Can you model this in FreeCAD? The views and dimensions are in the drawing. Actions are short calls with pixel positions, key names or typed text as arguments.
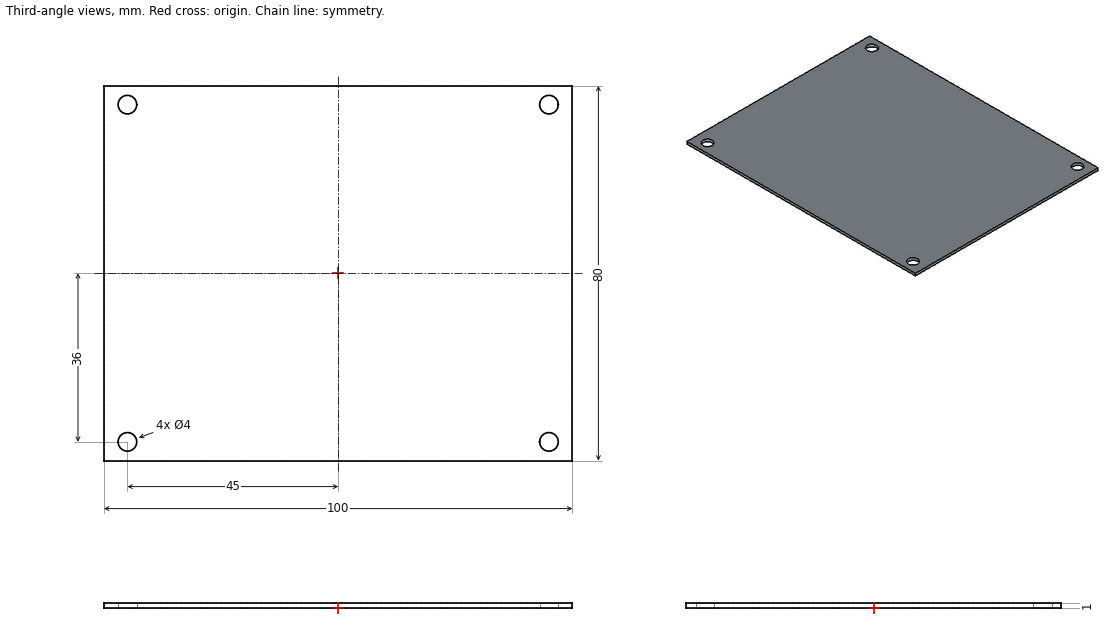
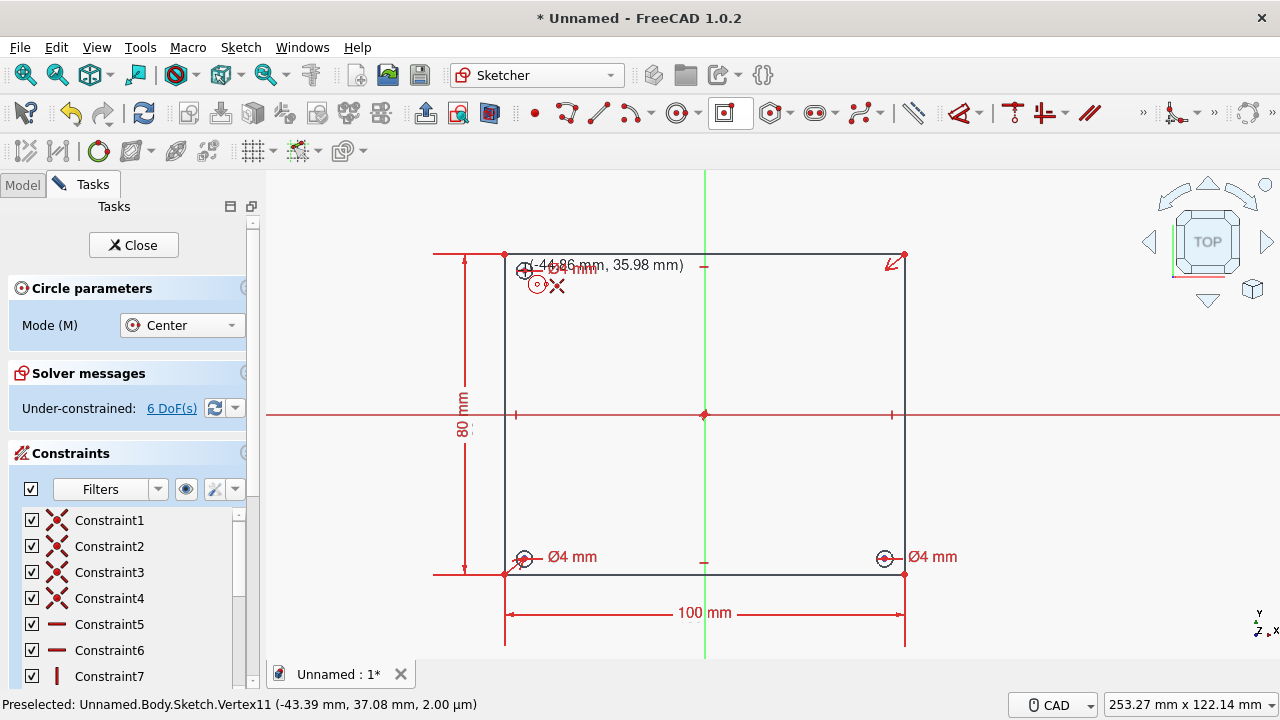
scroll(885, 270, up, 6)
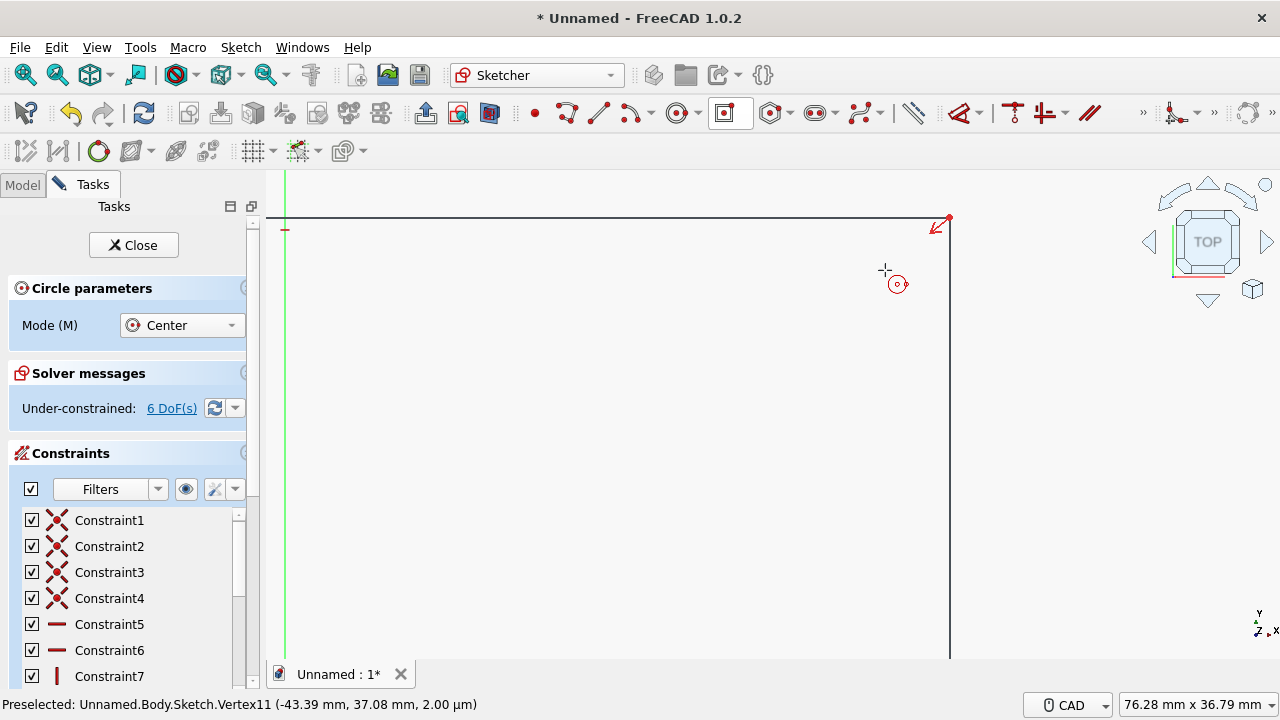
click(883, 271)
move(902, 252)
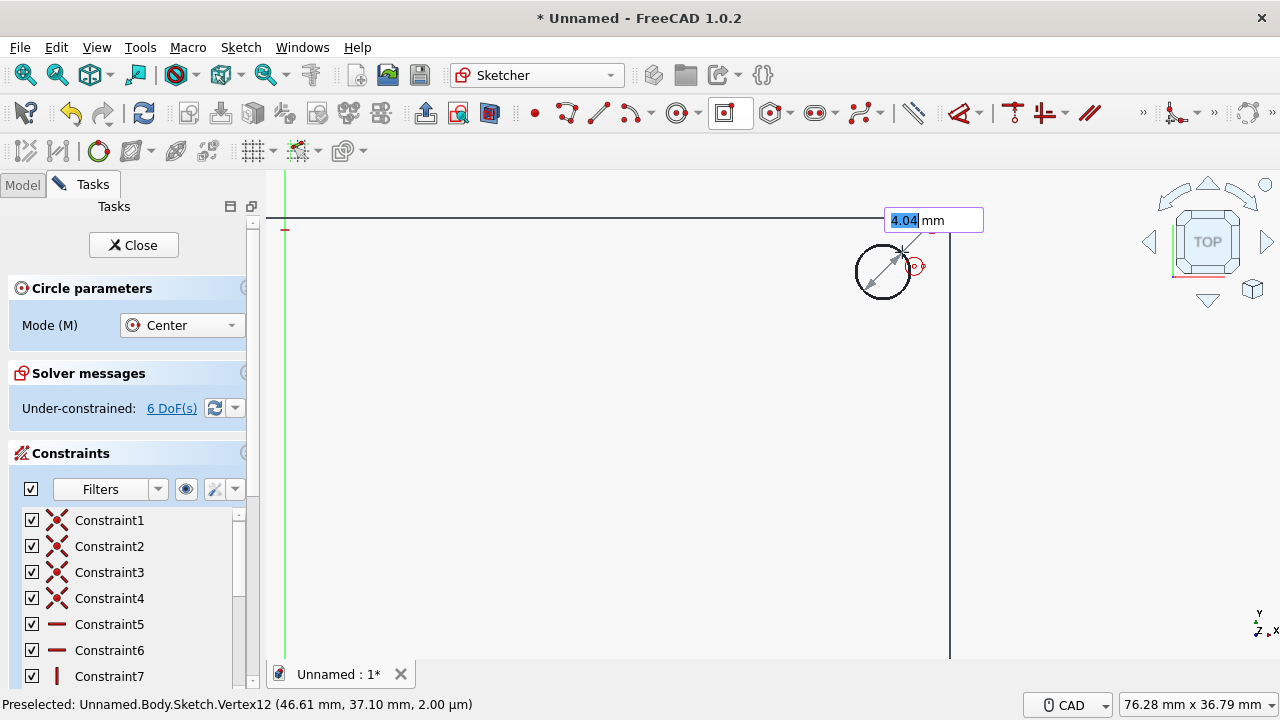
text(4)
key(Return)
key(Escape)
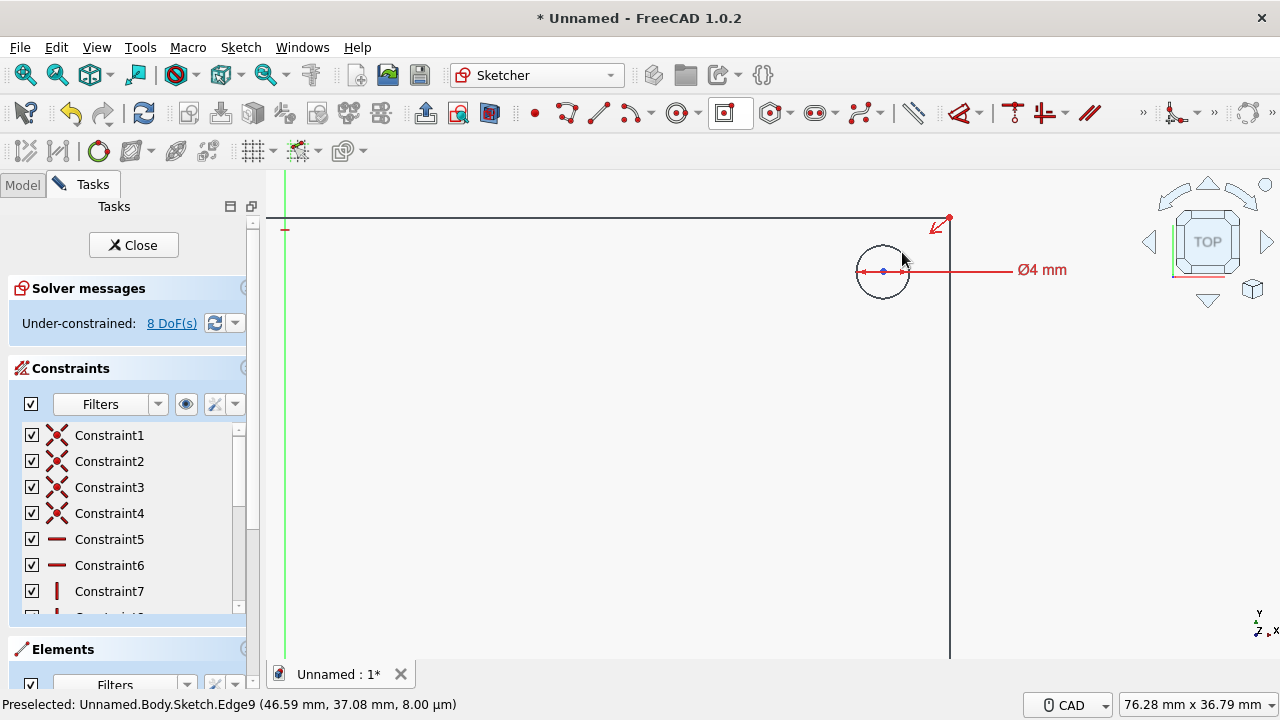
scroll(885, 270, down, 6)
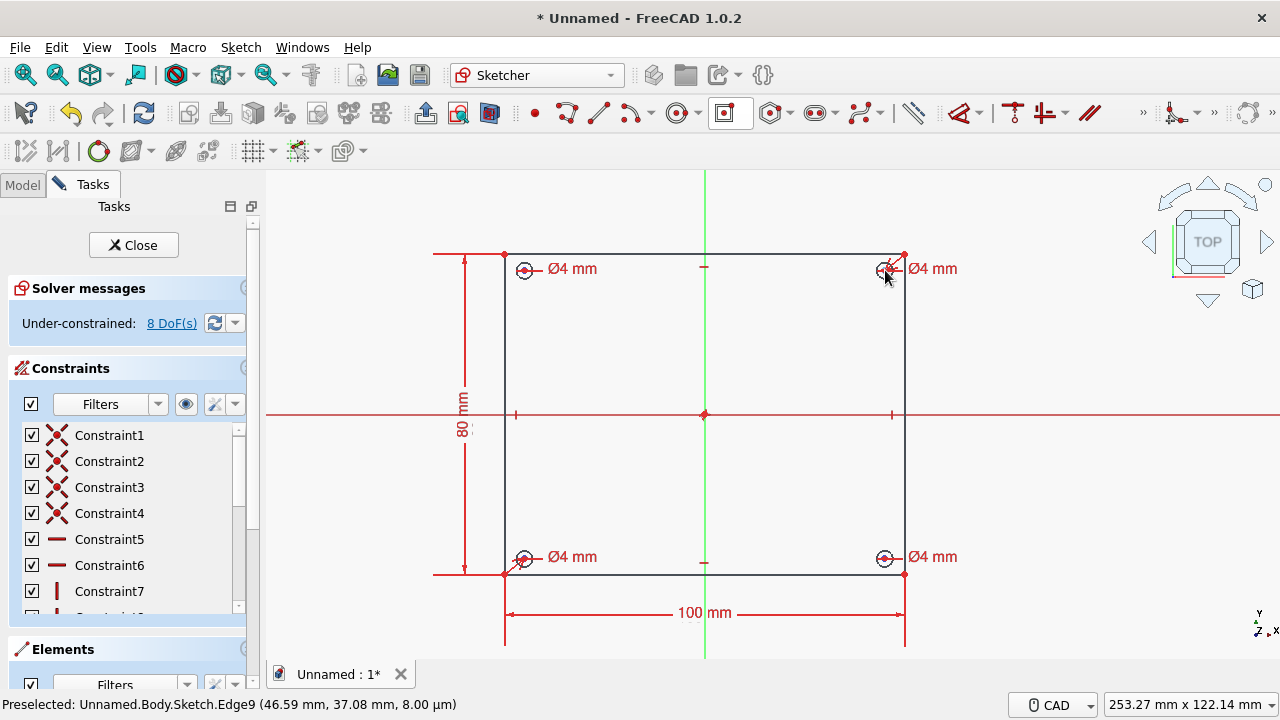
click(525, 559)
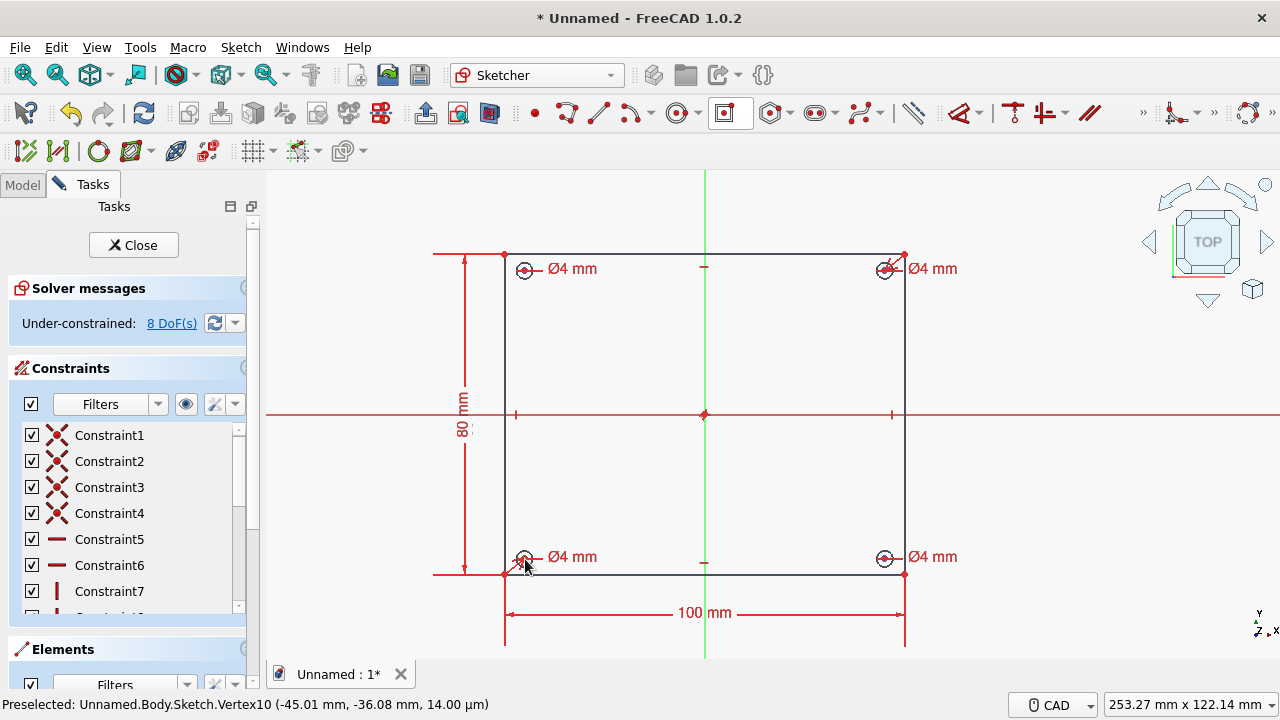
click(885, 559)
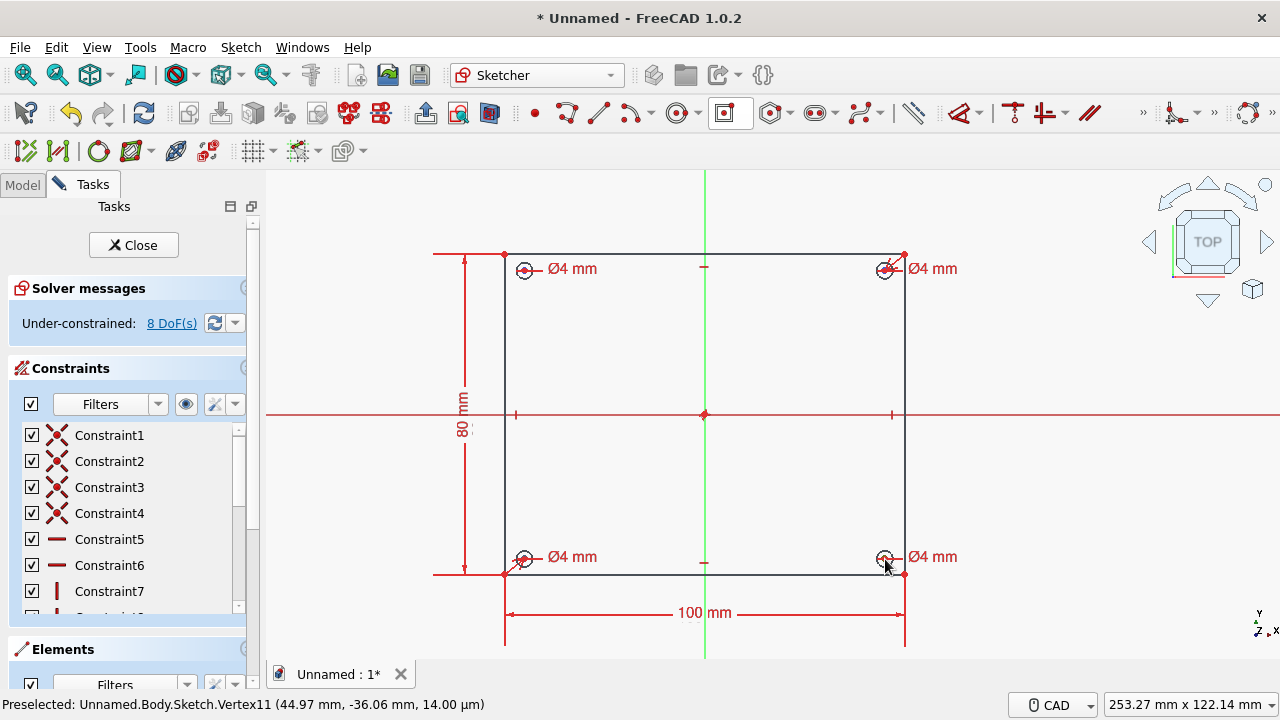
click(705, 538)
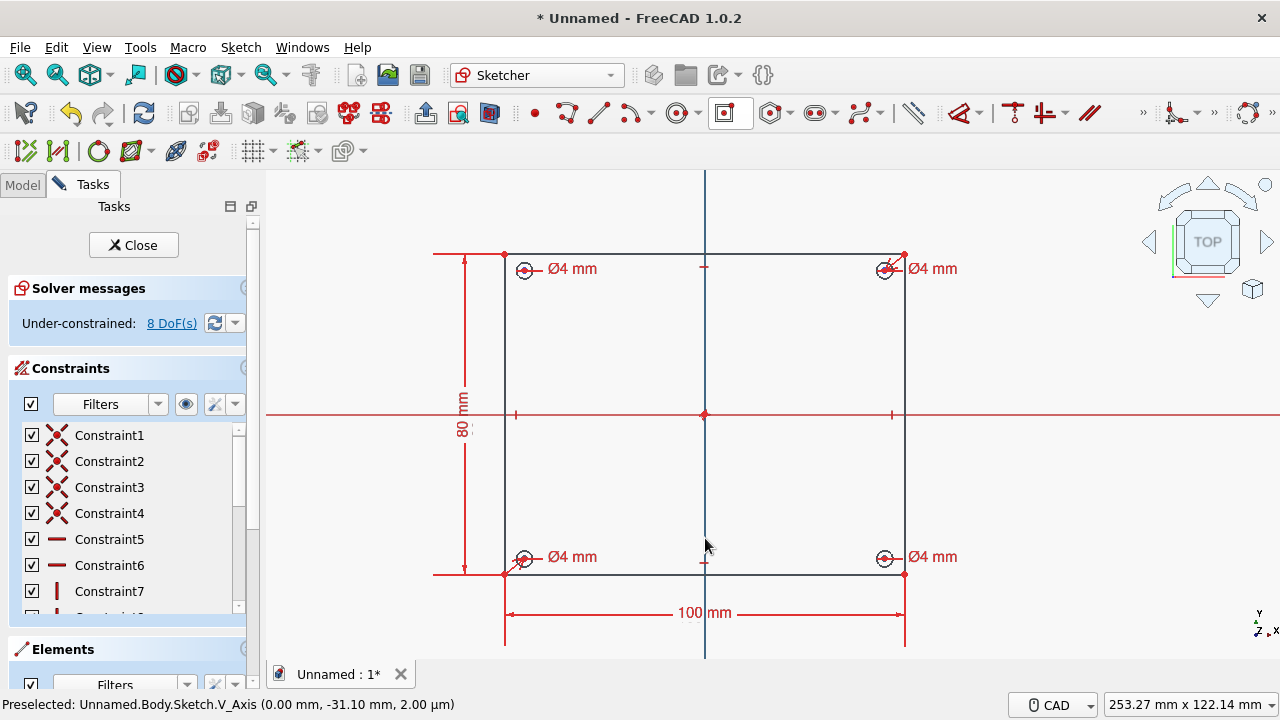
key(s)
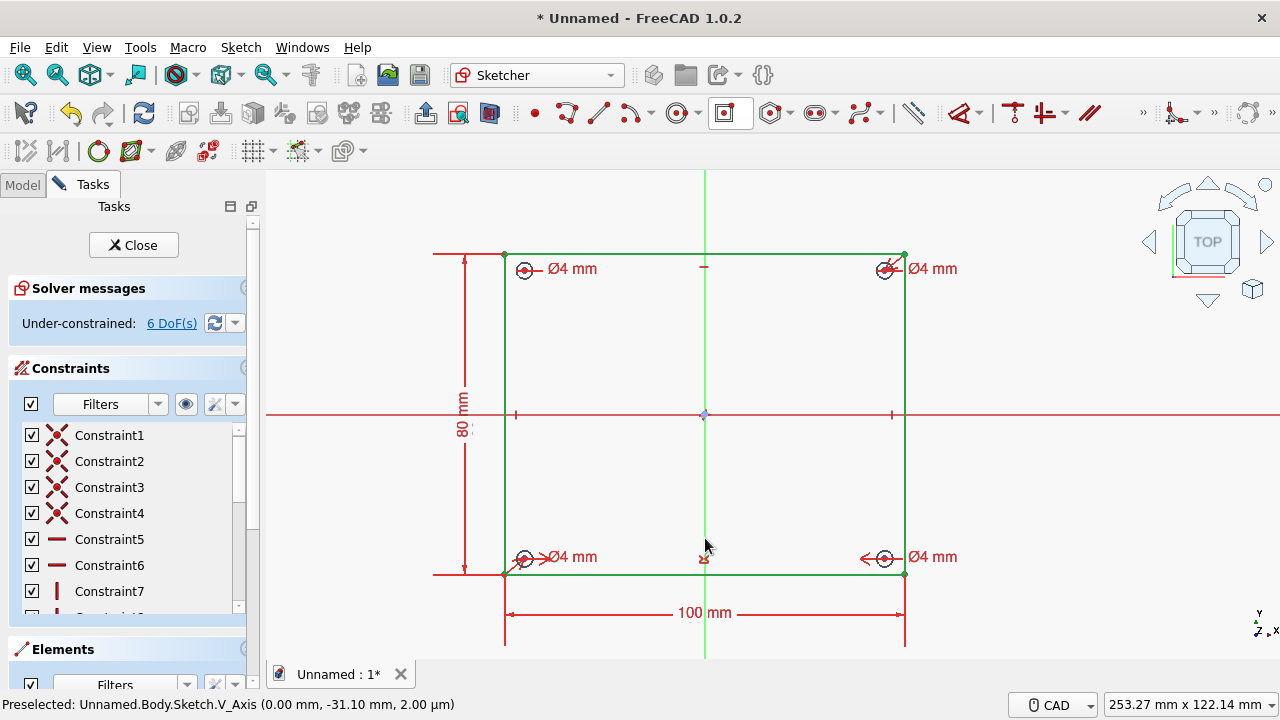
click(525, 559)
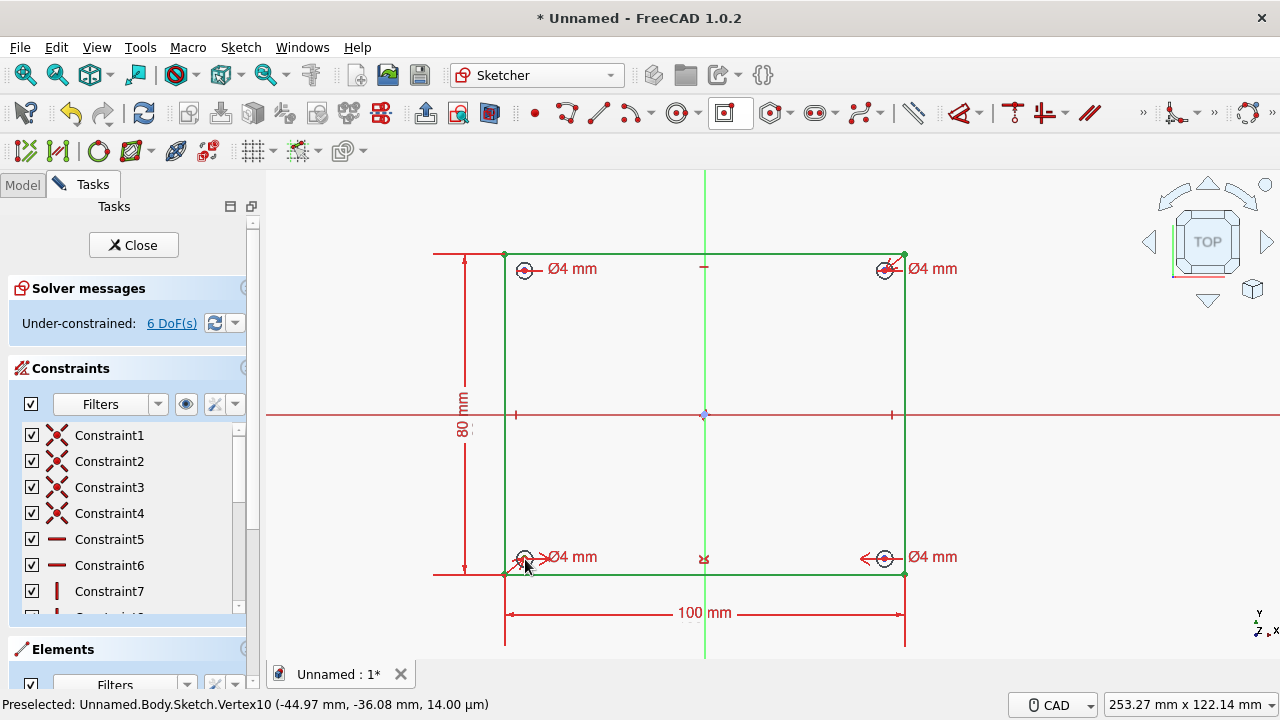
click(525, 271)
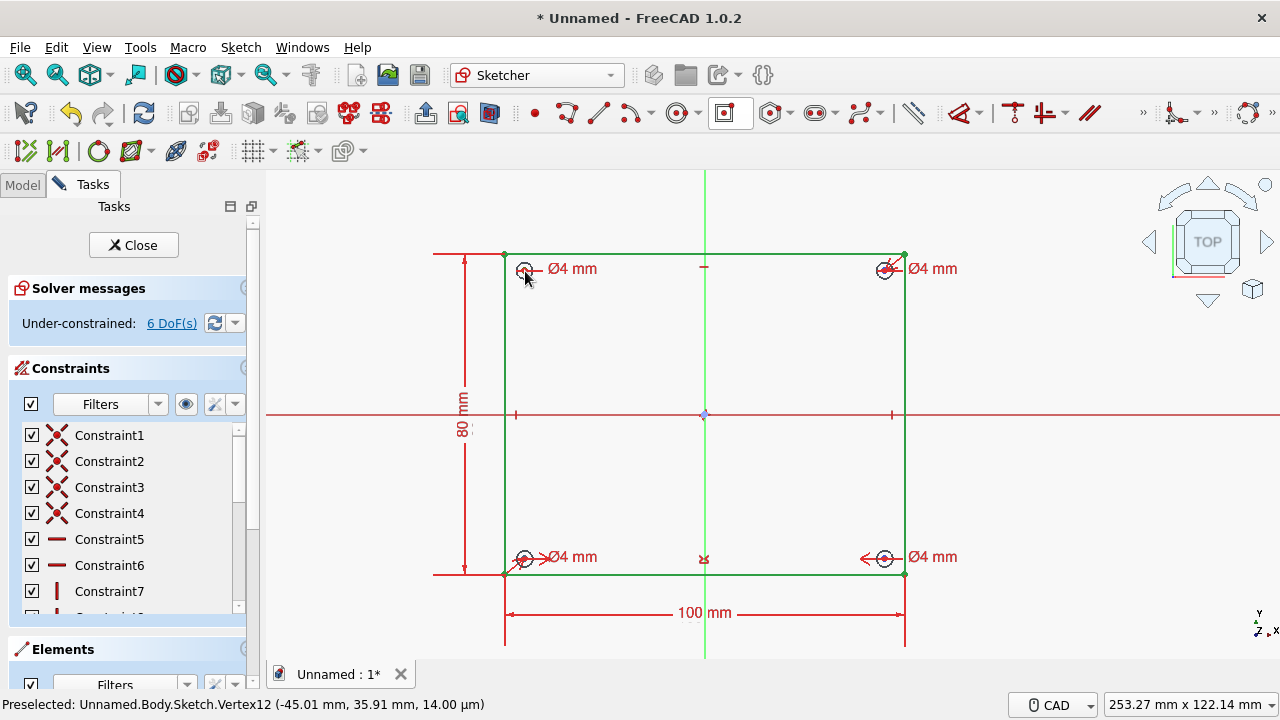
click(353, 414)